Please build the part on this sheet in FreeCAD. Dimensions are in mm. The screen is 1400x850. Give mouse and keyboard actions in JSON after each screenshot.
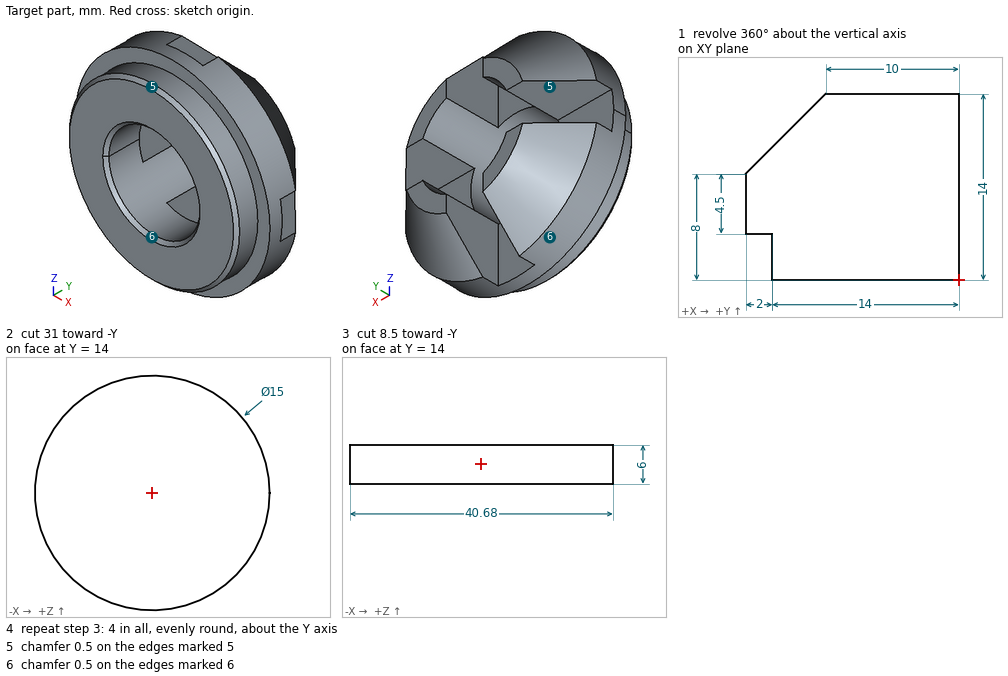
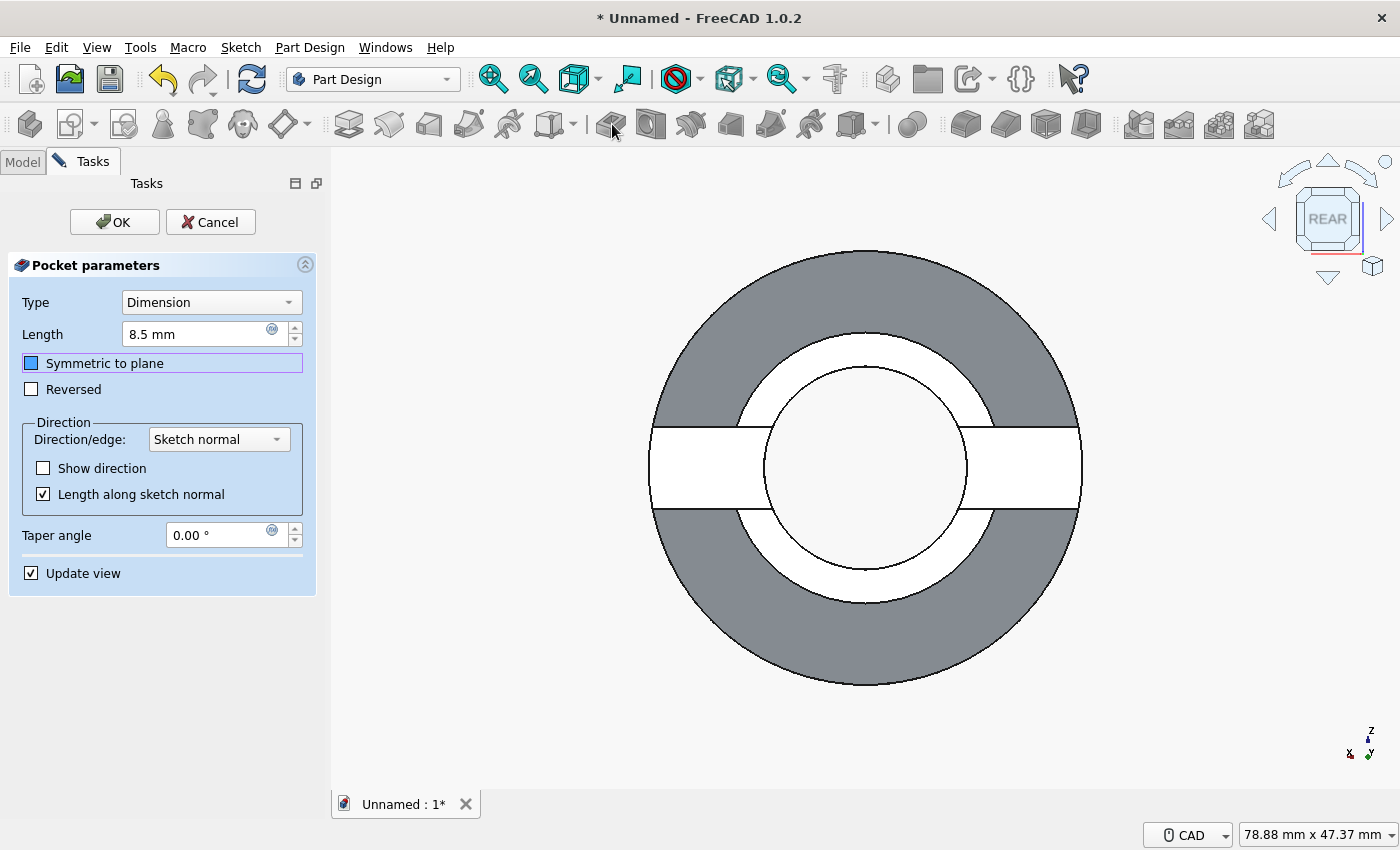
{"action": "left_click", "coordinate": [115, 222]}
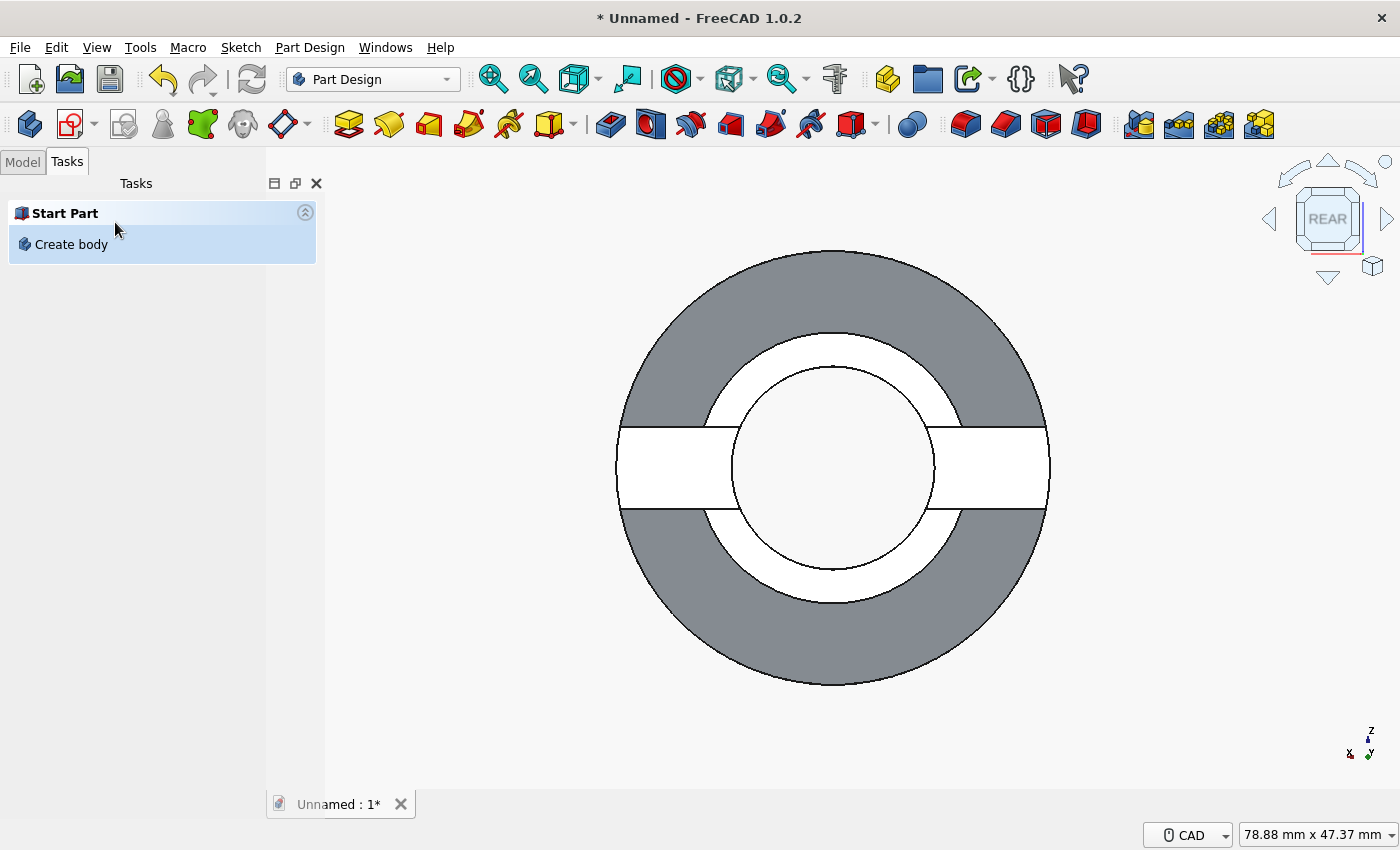
{"action": "left_click", "coordinate": [23, 161]}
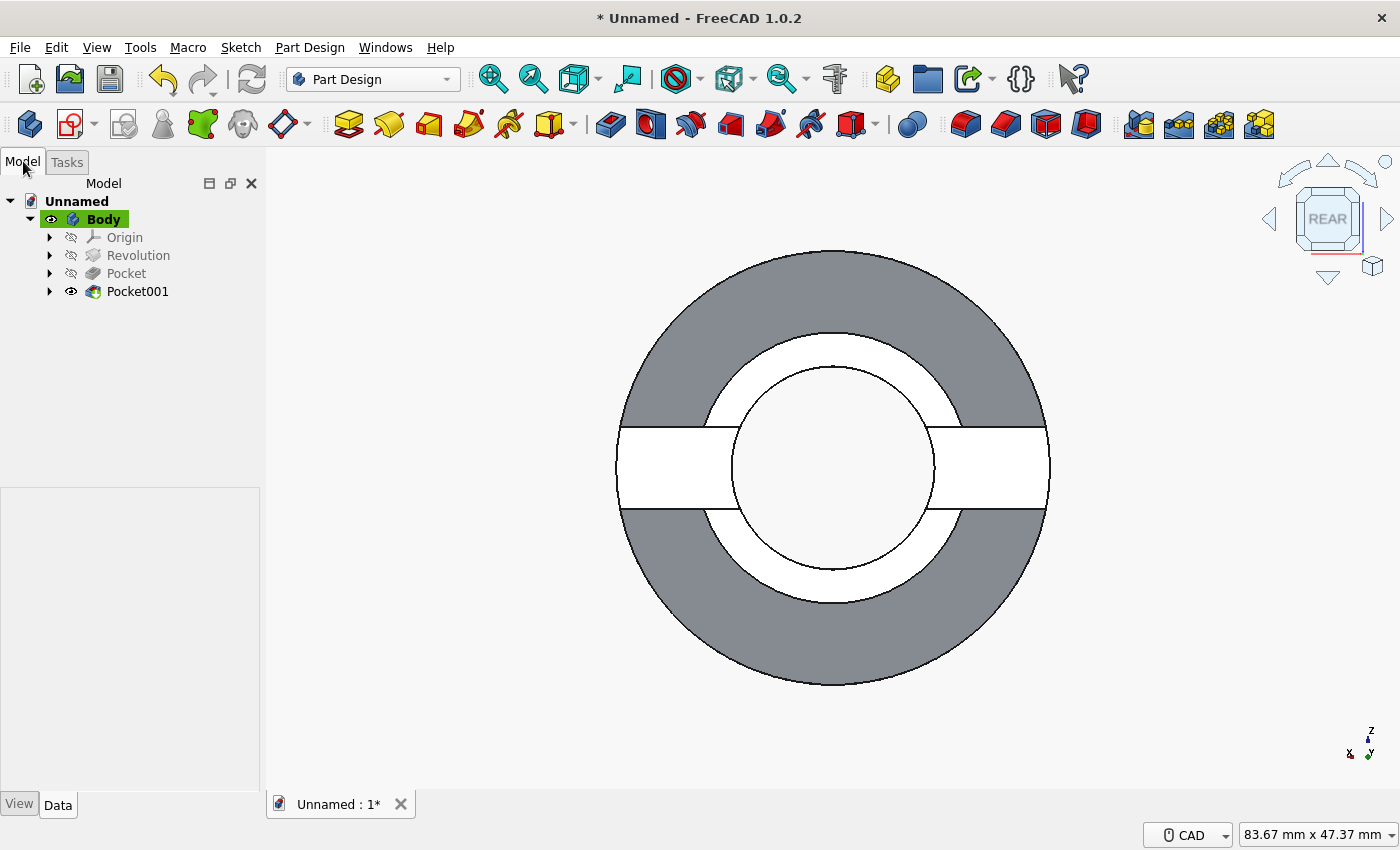
{"action": "left_click", "coordinate": [116, 291]}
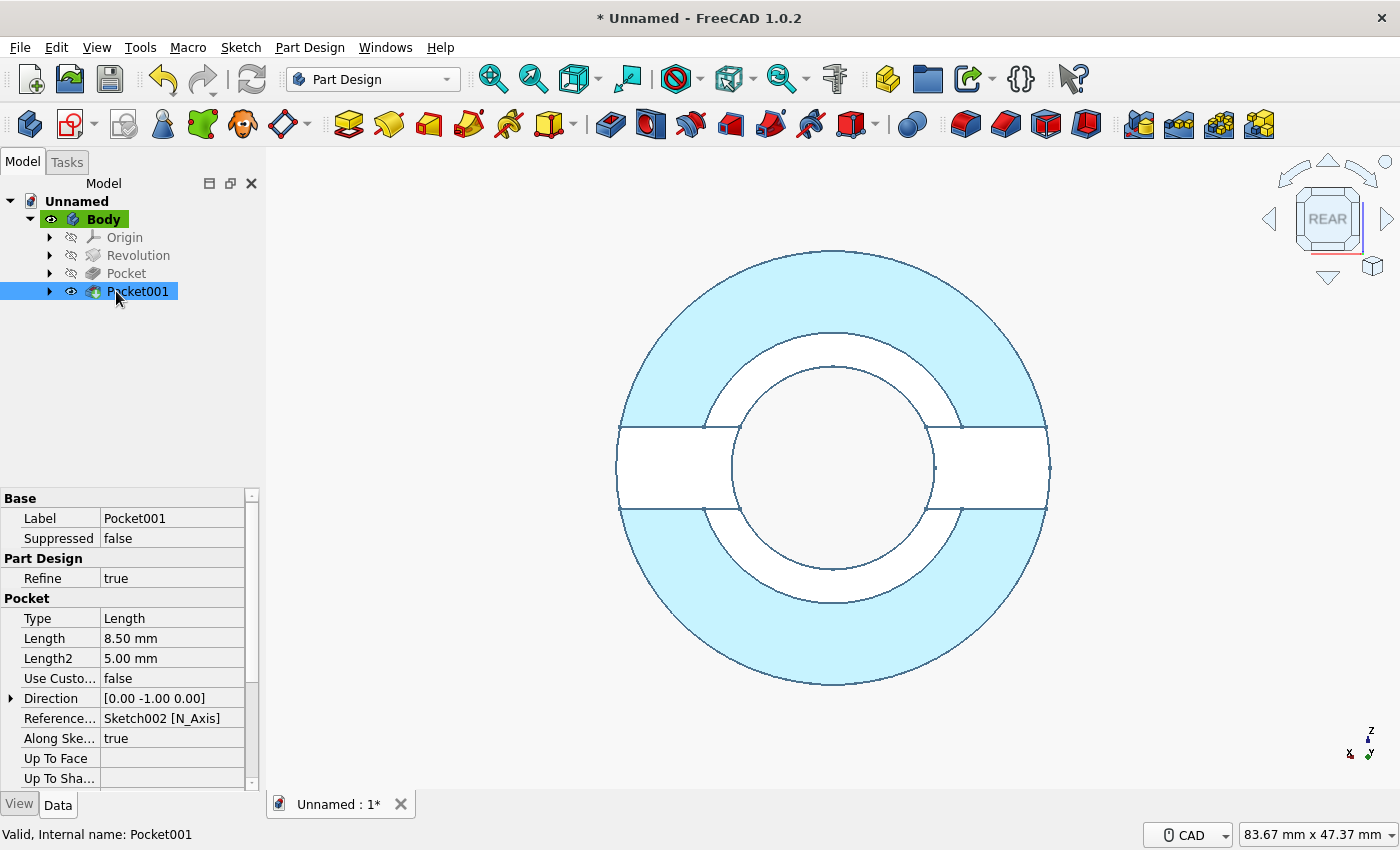
{"action": "left_click", "coordinate": [1220, 124]}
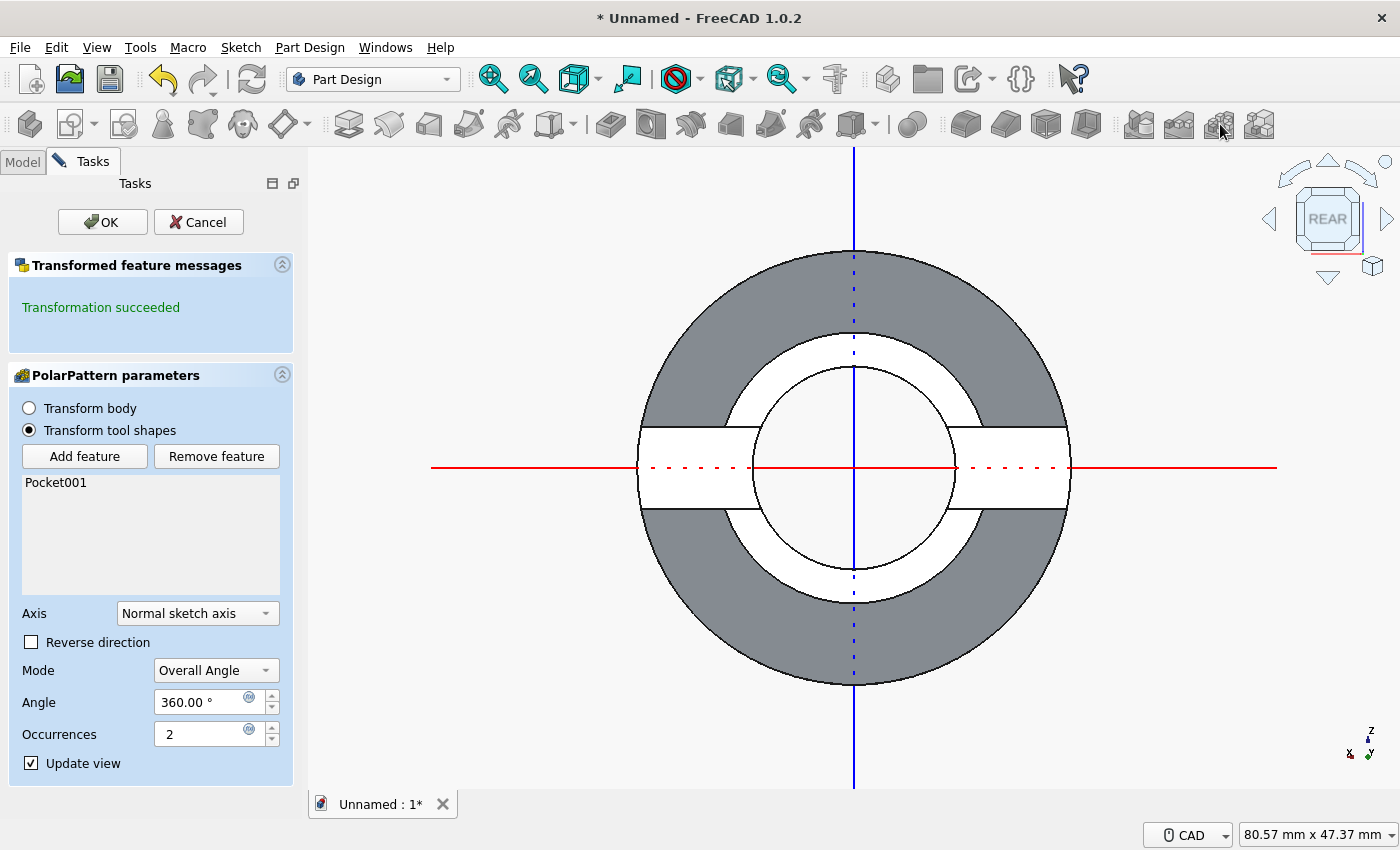
{"action": "left_click", "coordinate": [198, 614]}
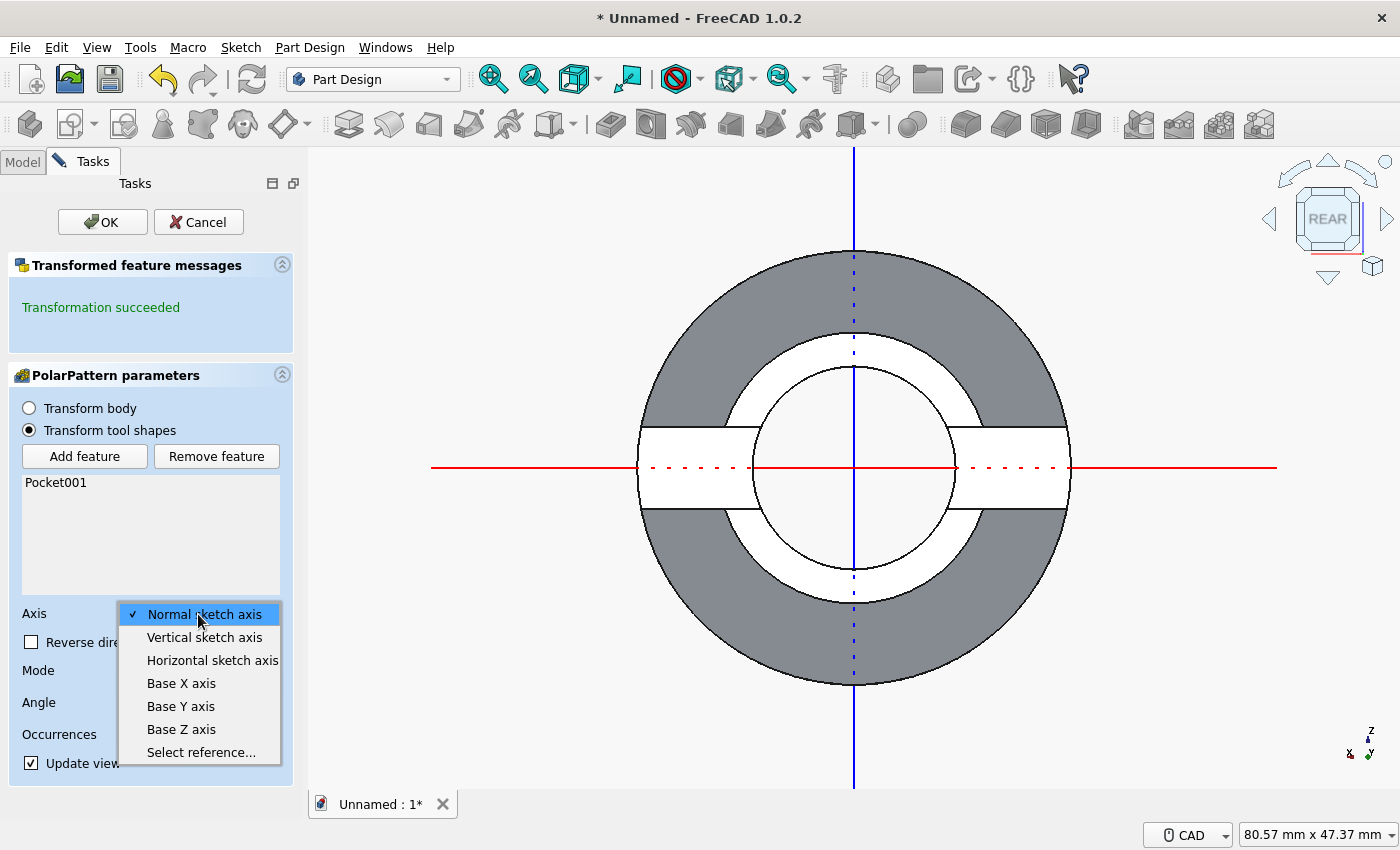
{"action": "left_click", "coordinate": [198, 706]}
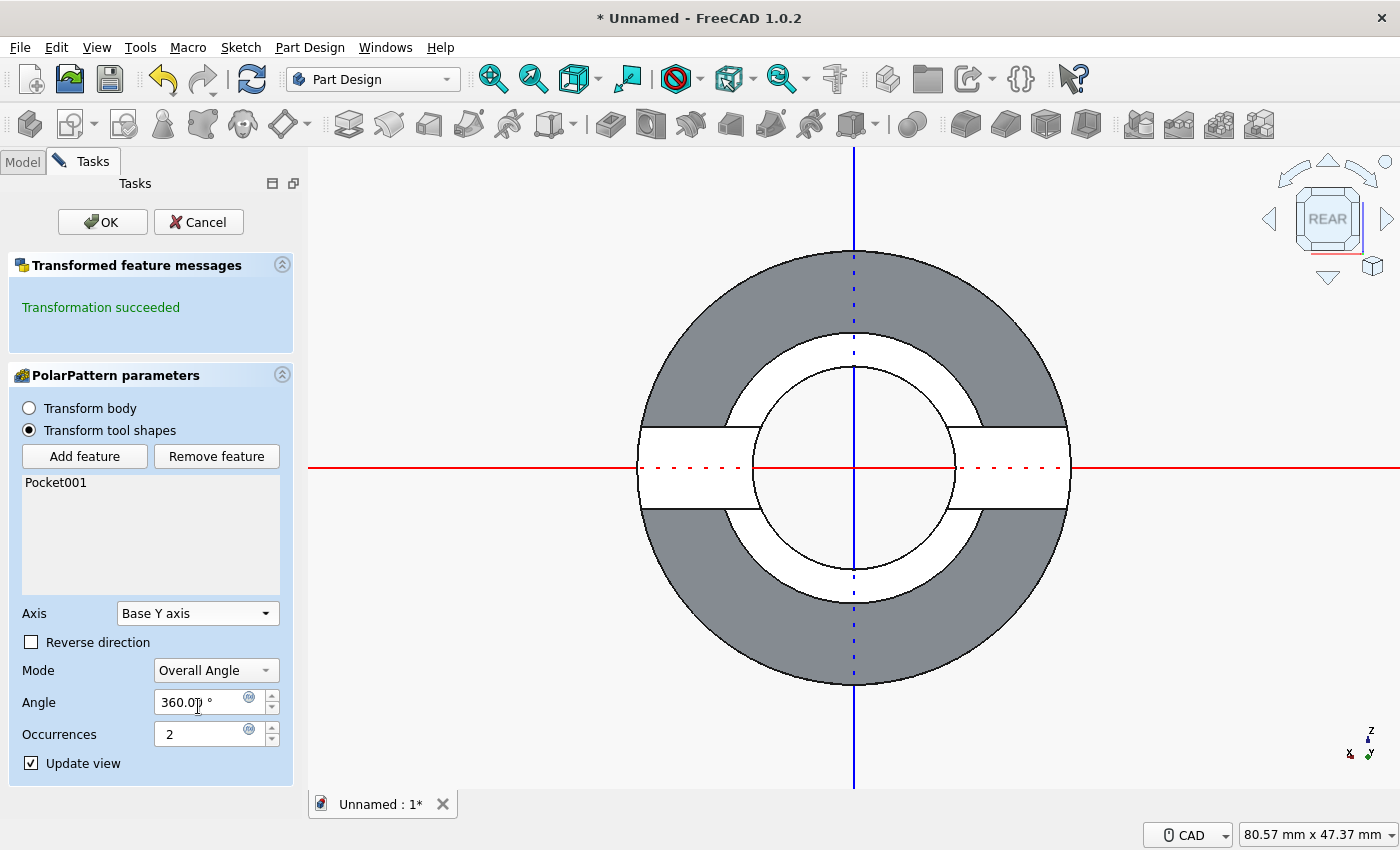
{"action": "triple_click", "coordinate": [209, 734]}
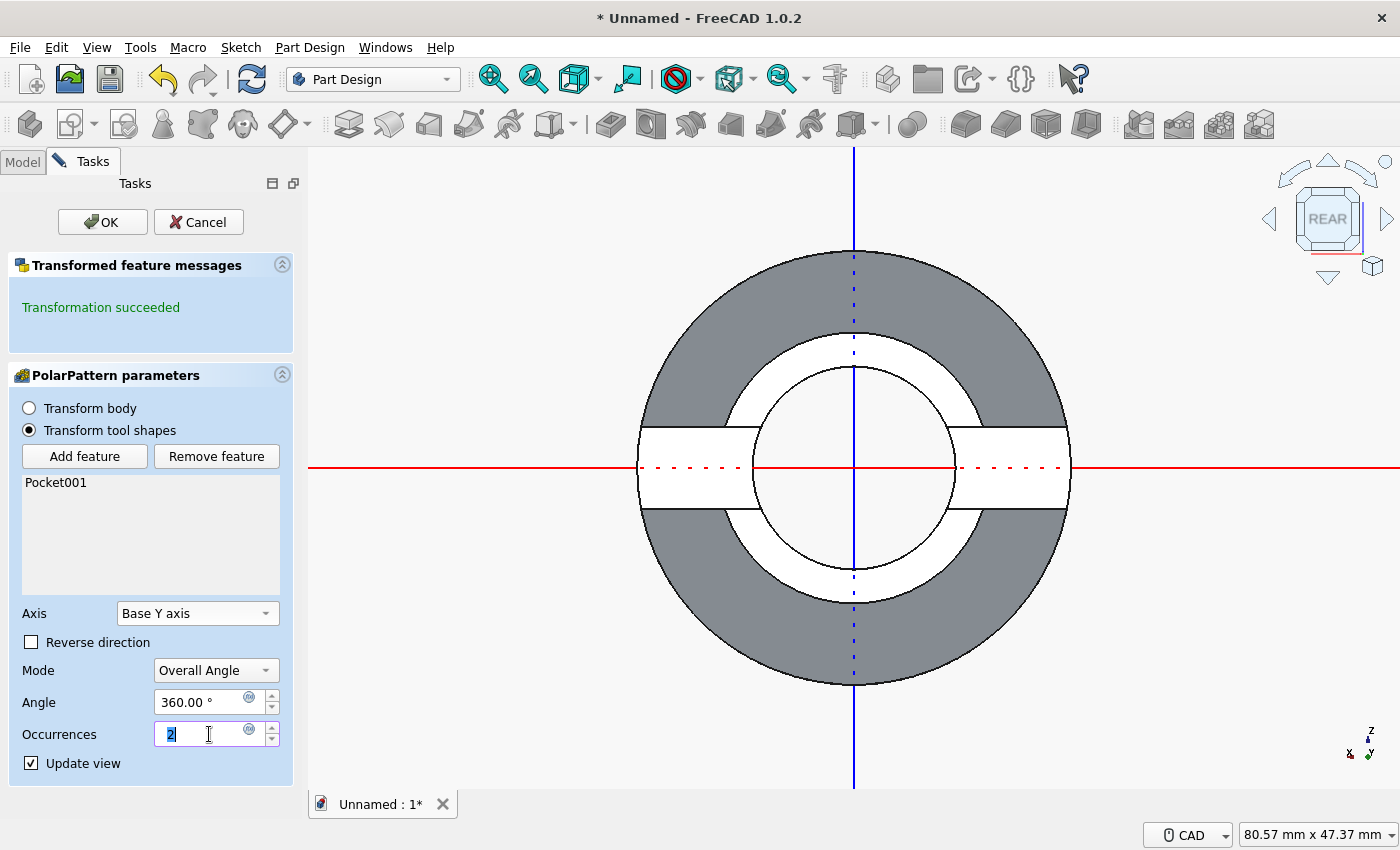
{"action": "type", "text": "4"}
{"action": "key", "text": "Tab"}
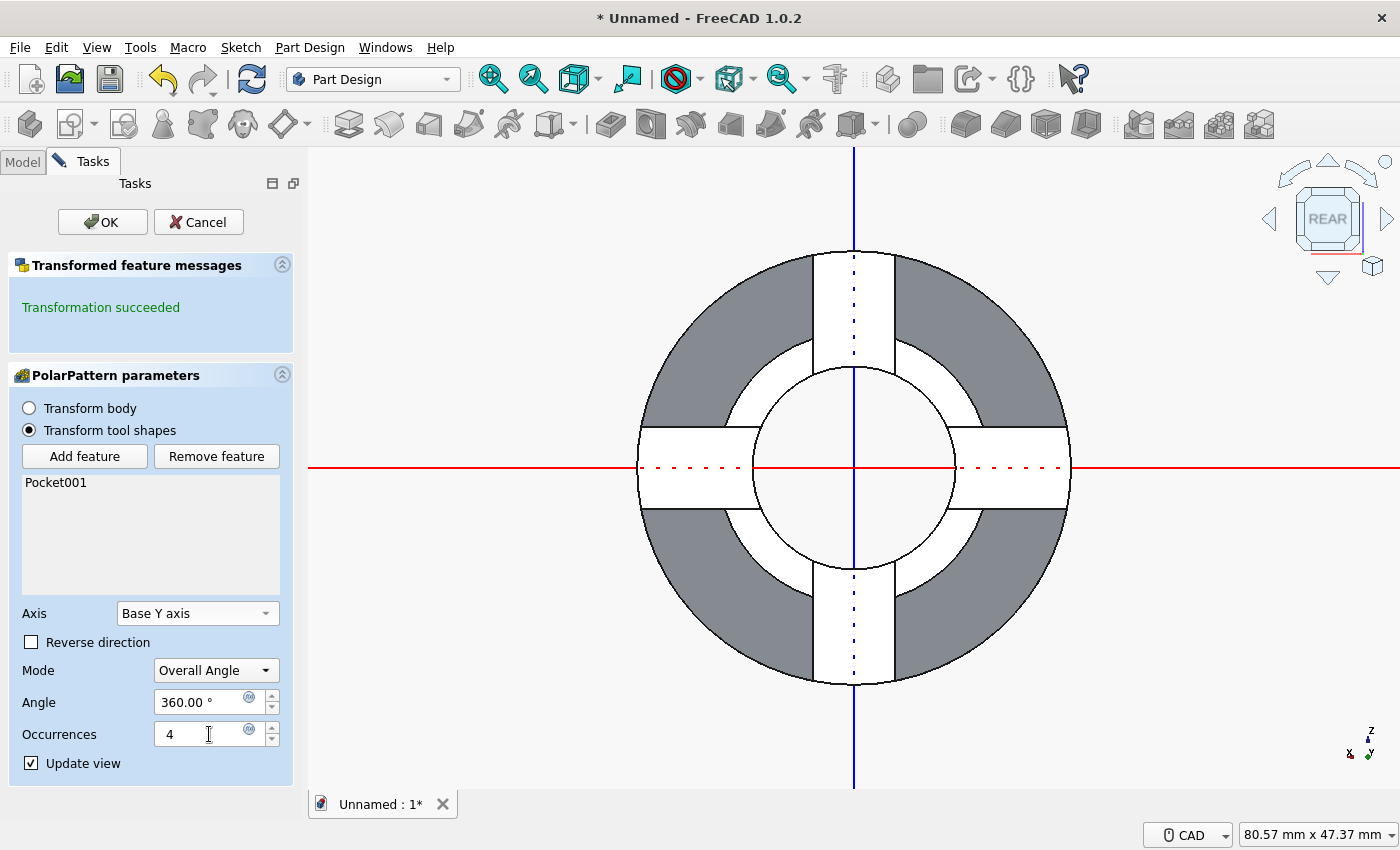
{"action": "left_click", "coordinate": [103, 222]}